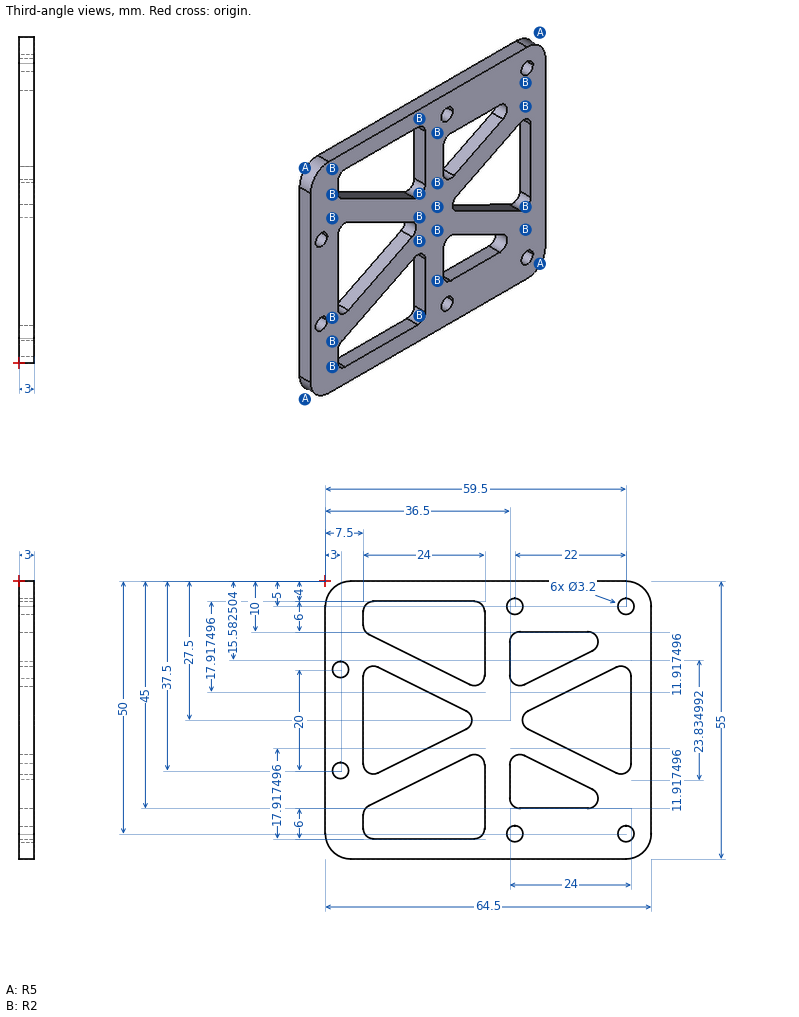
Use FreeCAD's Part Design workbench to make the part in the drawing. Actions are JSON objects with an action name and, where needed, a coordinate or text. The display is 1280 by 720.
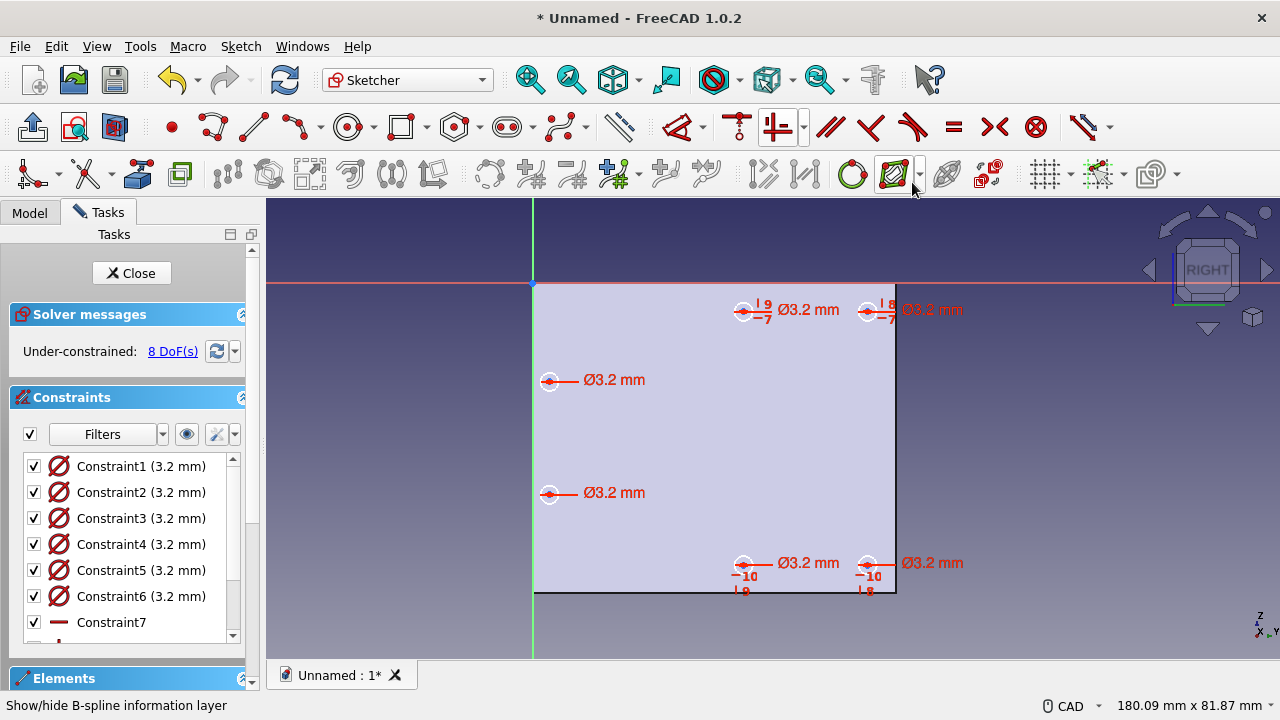
{"action": "left_click", "coordinate": [550, 495]}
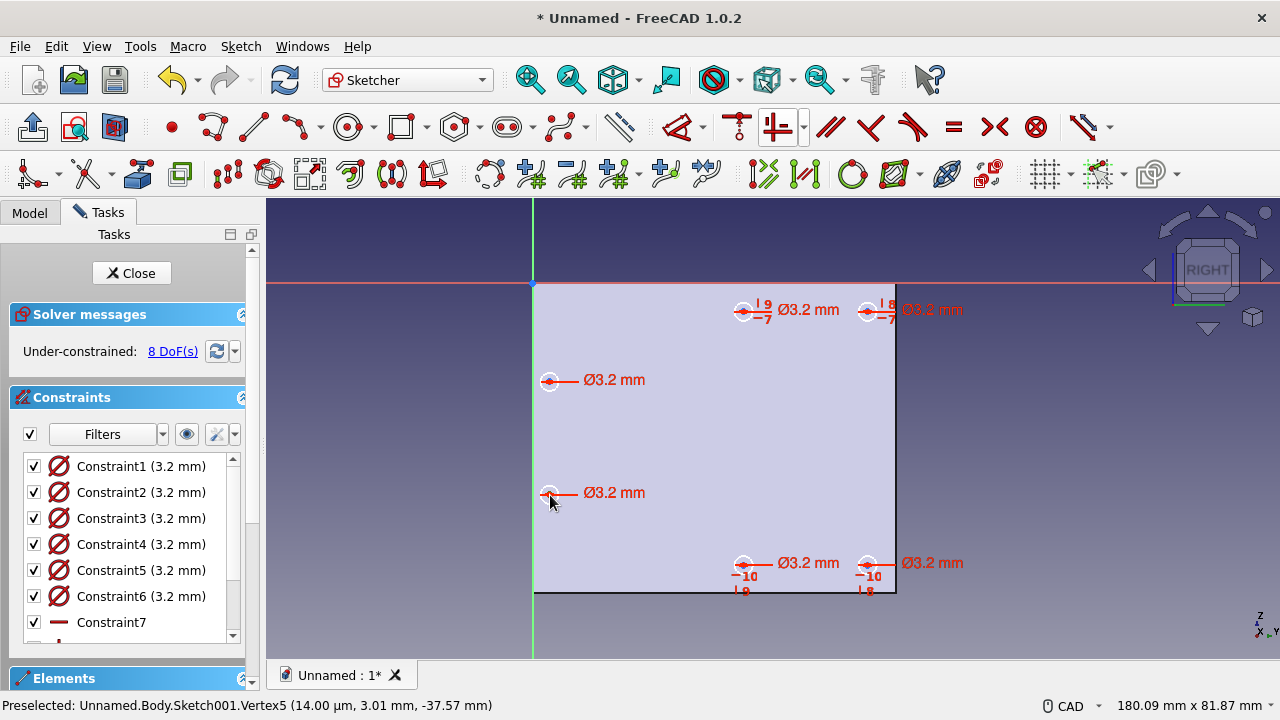
{"action": "left_click", "coordinate": [550, 382]}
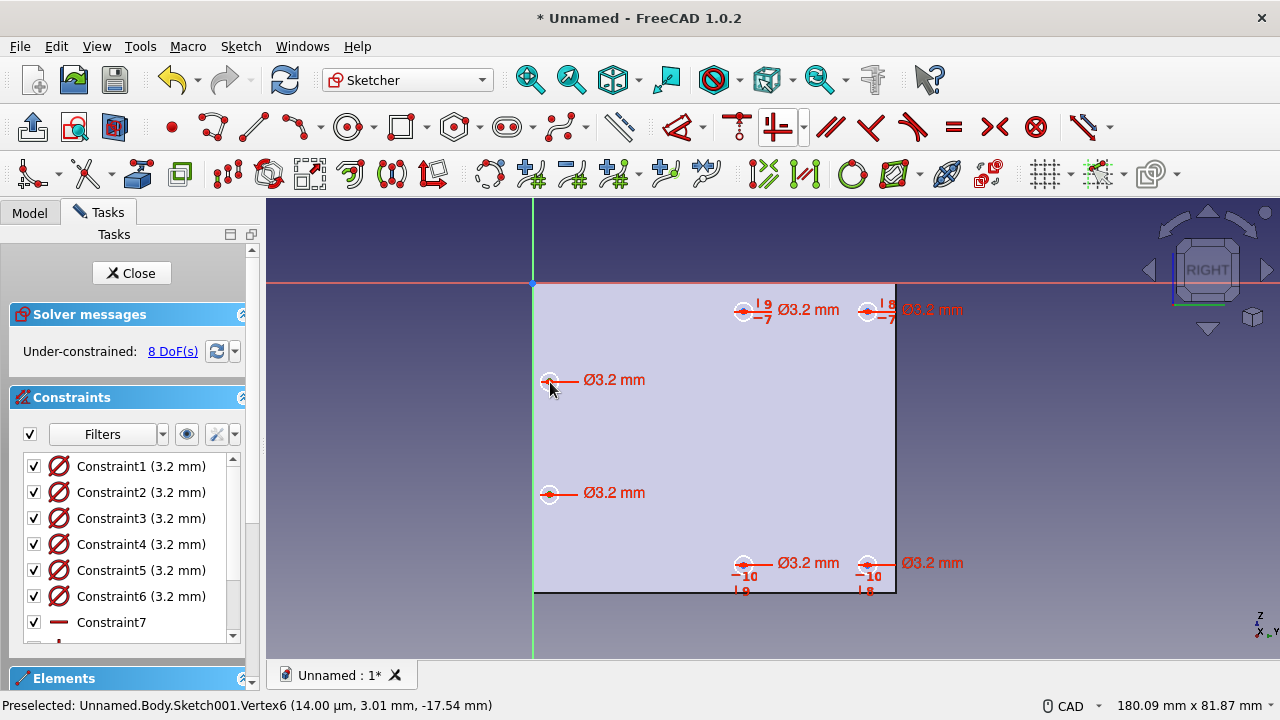
{"action": "left_click", "coordinate": [804, 128]}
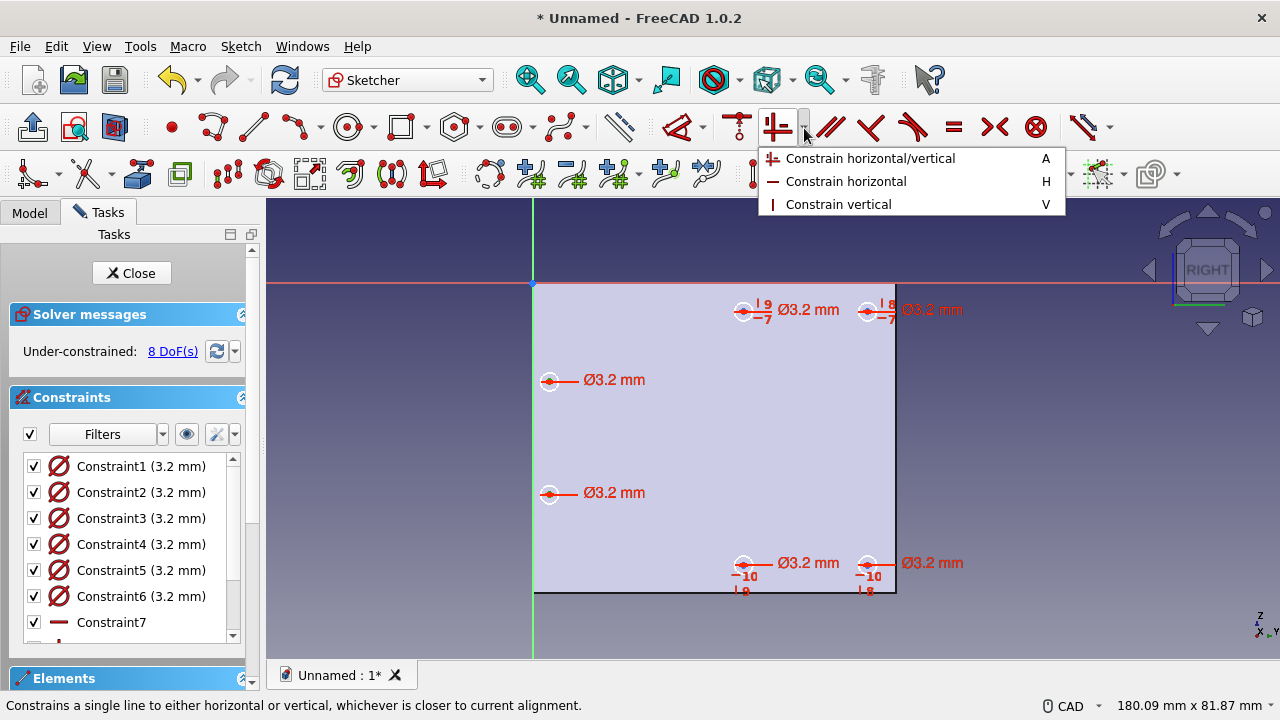
{"action": "left_click", "coordinate": [912, 204]}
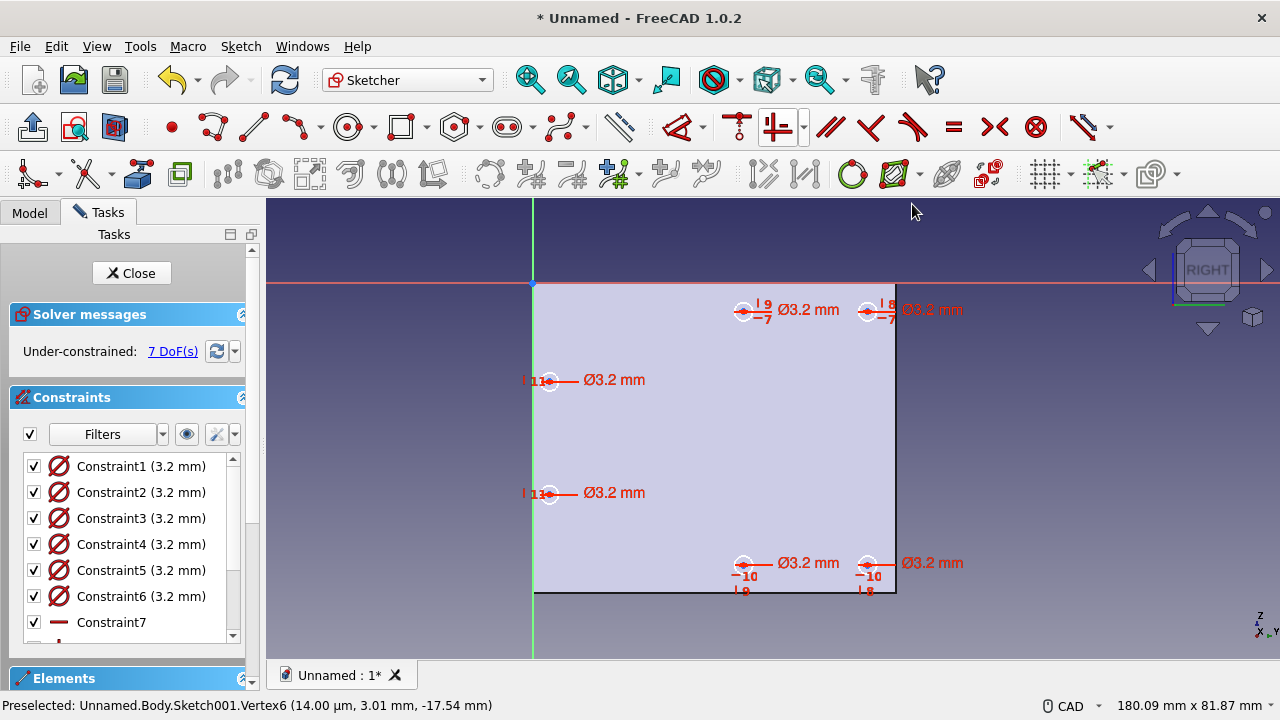
{"action": "left_click", "coordinate": [676, 128]}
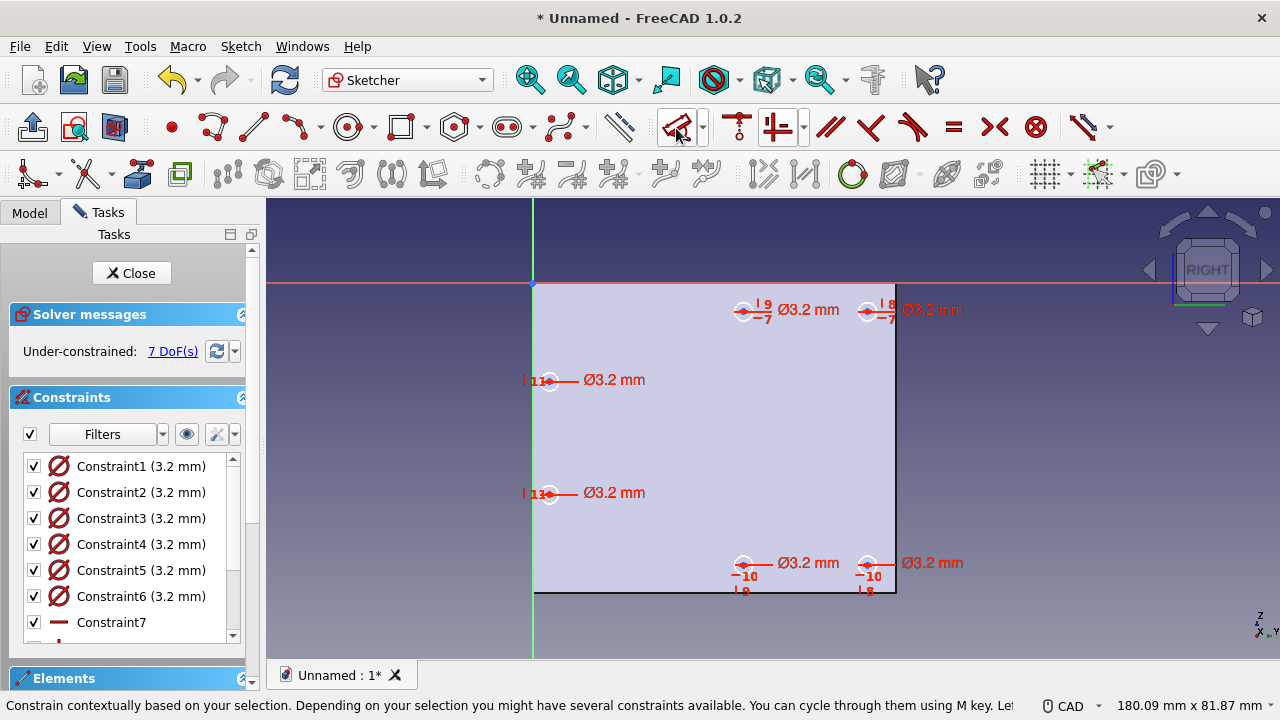
{"action": "scroll", "coordinate": [868, 312], "scroll_direction": "up", "scroll_amount": 2}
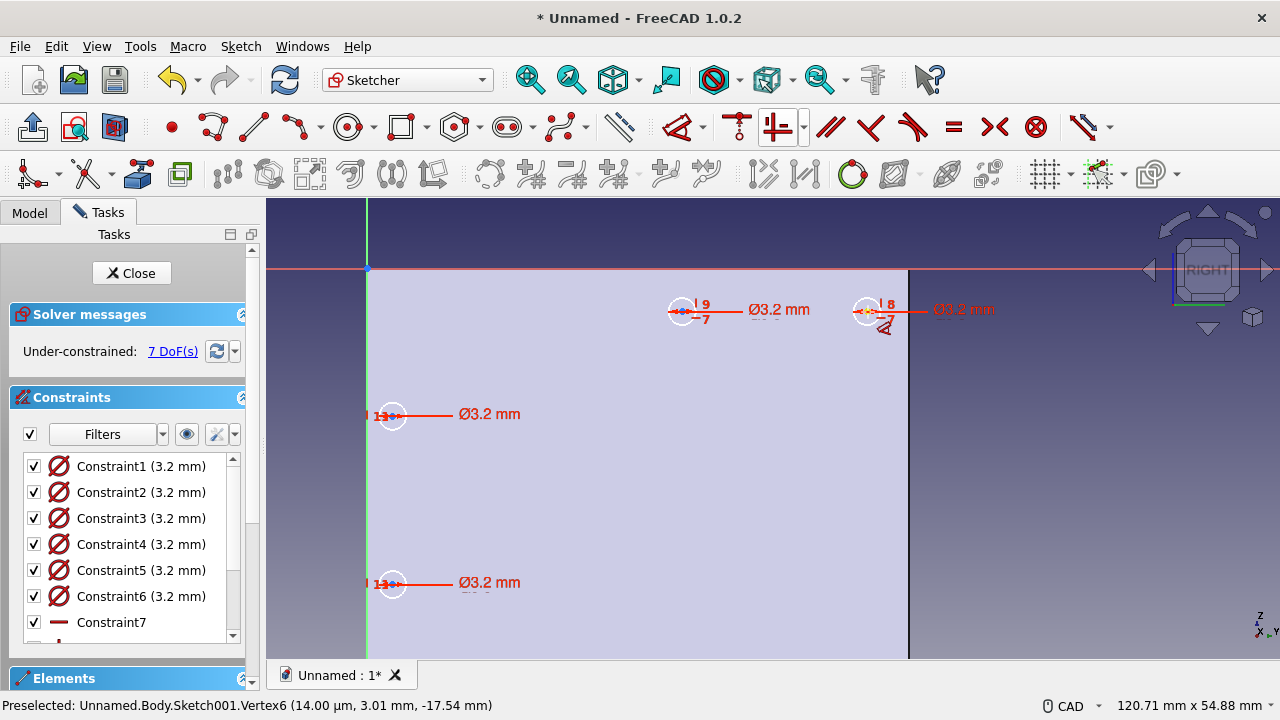
{"action": "left_click", "coordinate": [867, 312]}
{"action": "left_click", "coordinate": [333, 290]}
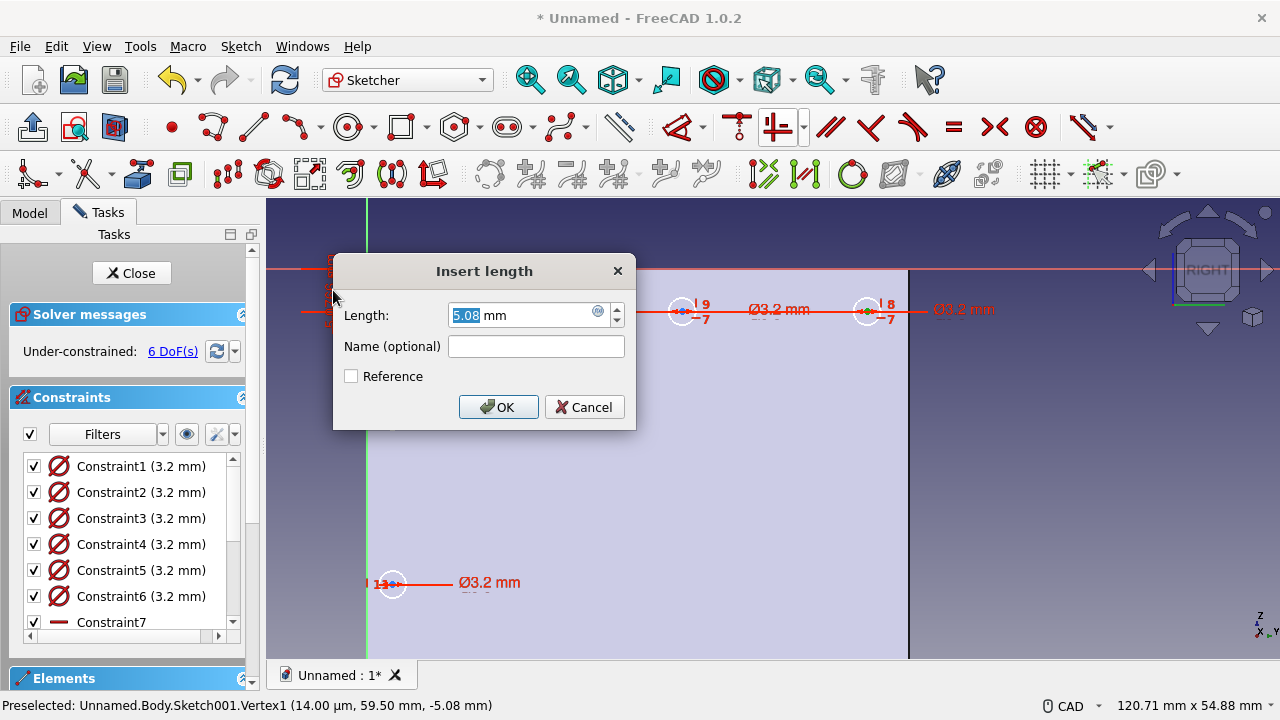
{"action": "type", "text": "5"}
{"action": "key", "text": "Return"}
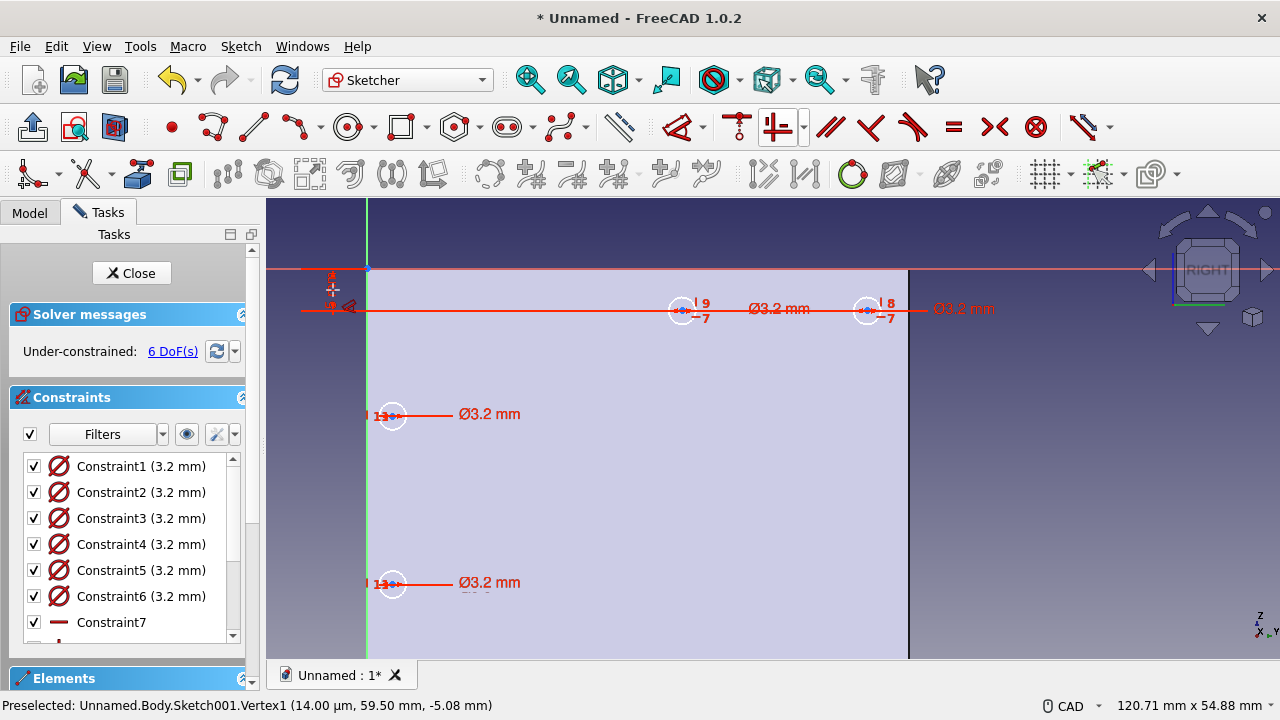
{"action": "scroll", "coordinate": [393, 585], "scroll_direction": "up", "scroll_amount": 3}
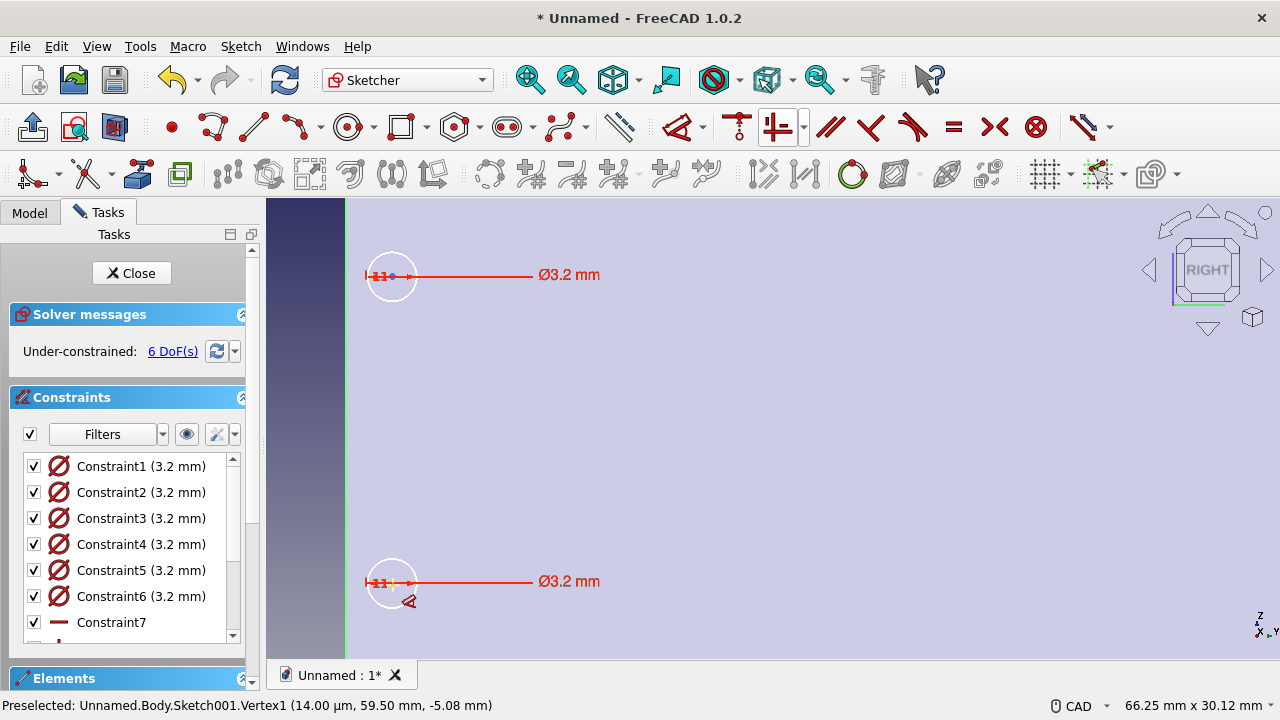
{"action": "left_click", "coordinate": [392, 583]}
{"action": "left_click", "coordinate": [369, 617]}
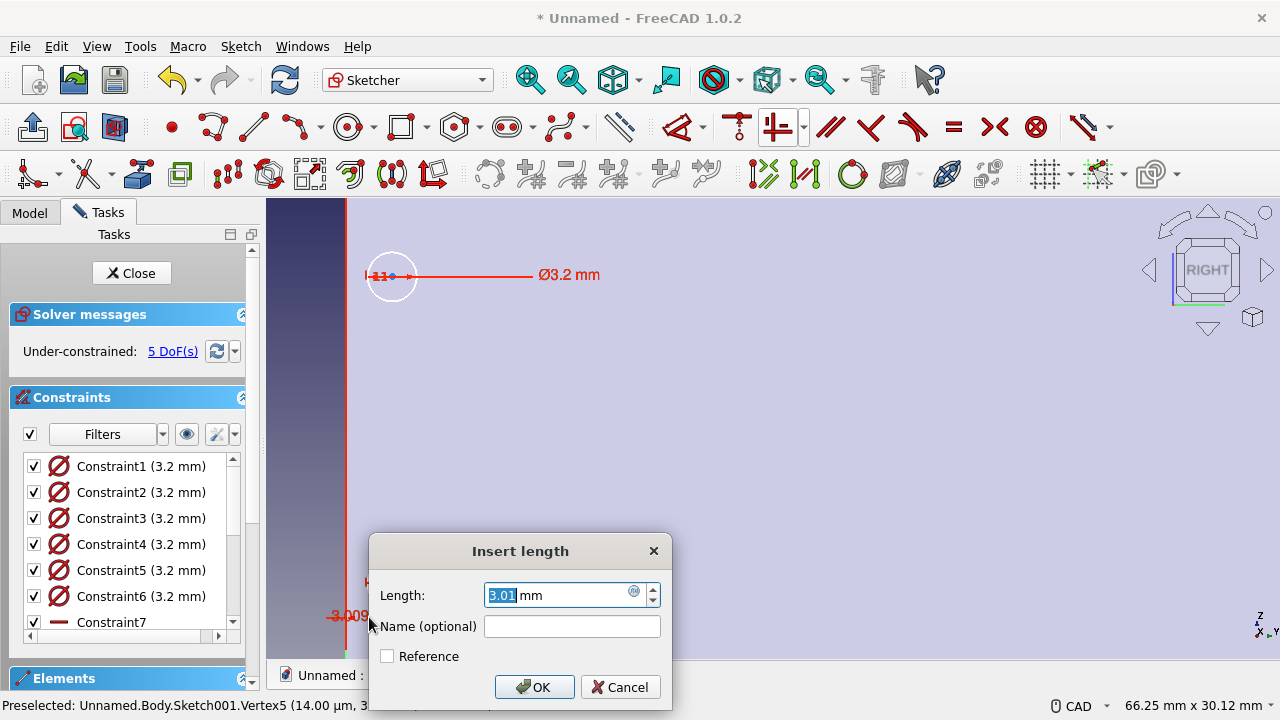
{"action": "type", "text": "3"}
{"action": "key", "text": "Return"}